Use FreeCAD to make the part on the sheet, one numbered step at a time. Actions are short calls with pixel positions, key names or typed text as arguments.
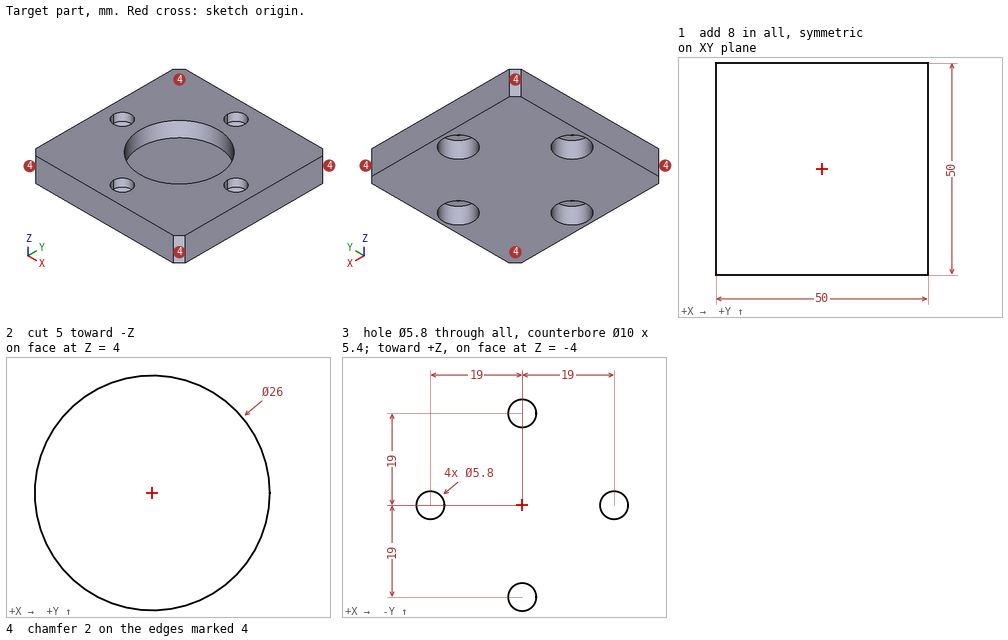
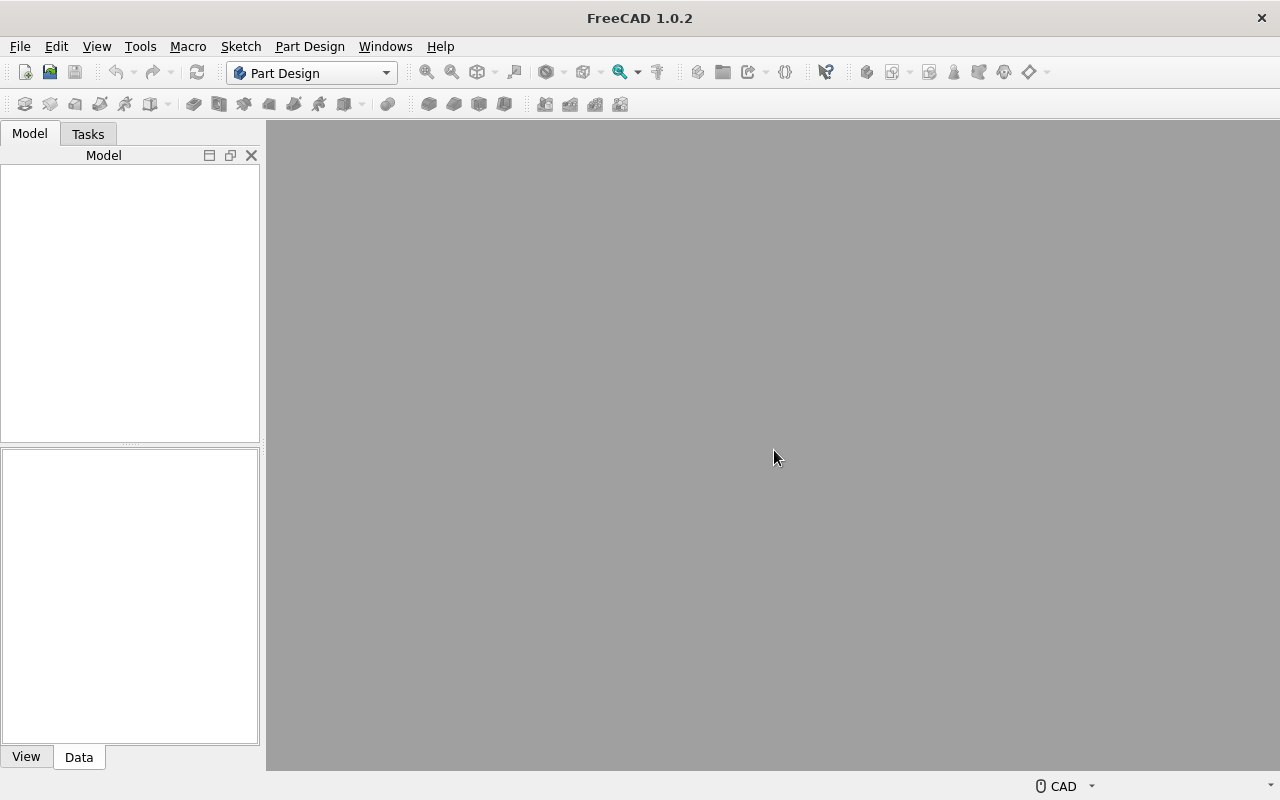
click(25, 72)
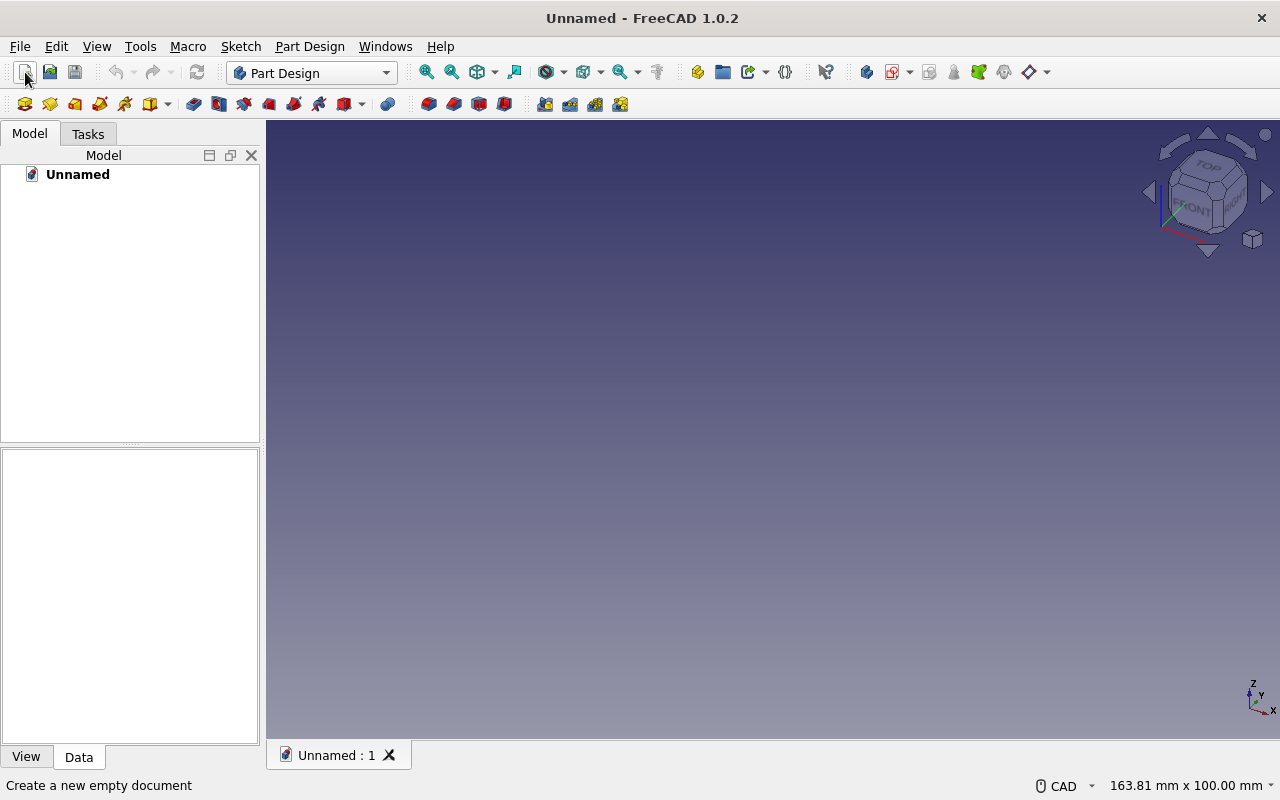
click(892, 72)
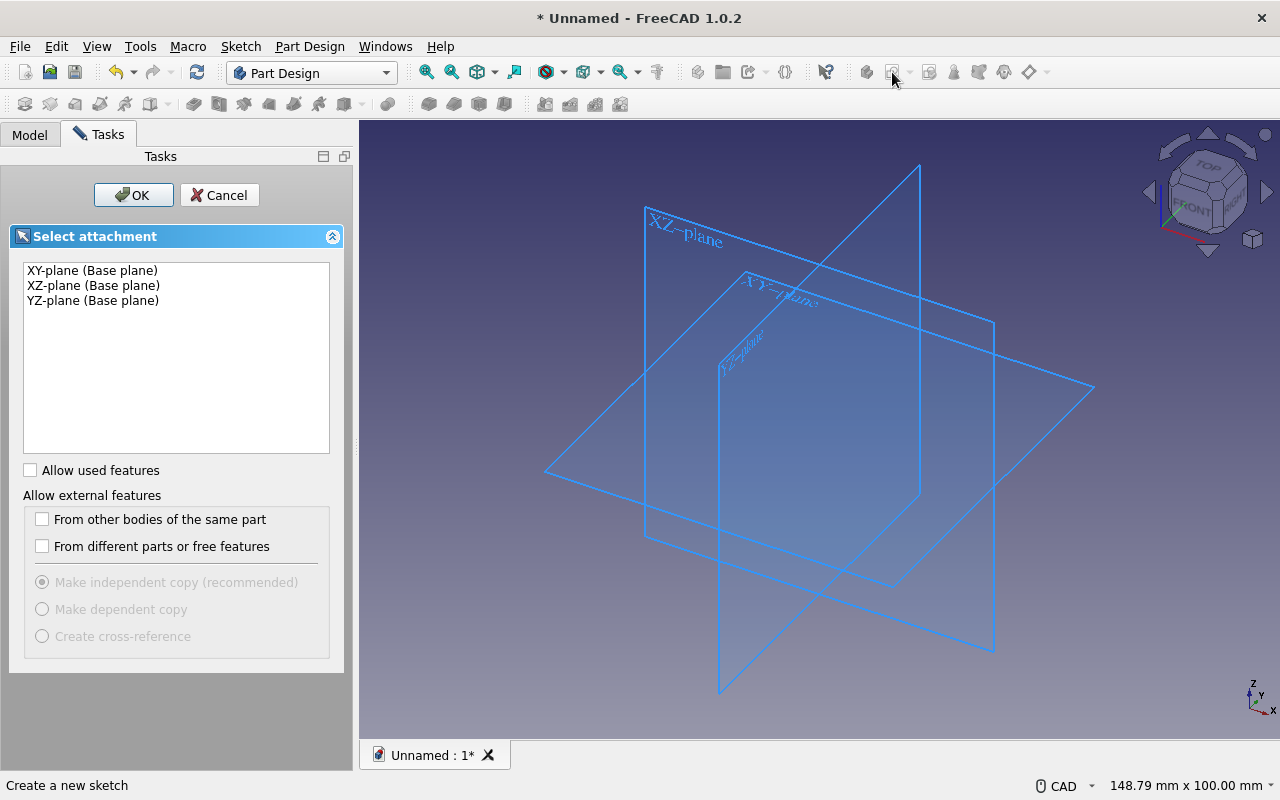
click(84, 270)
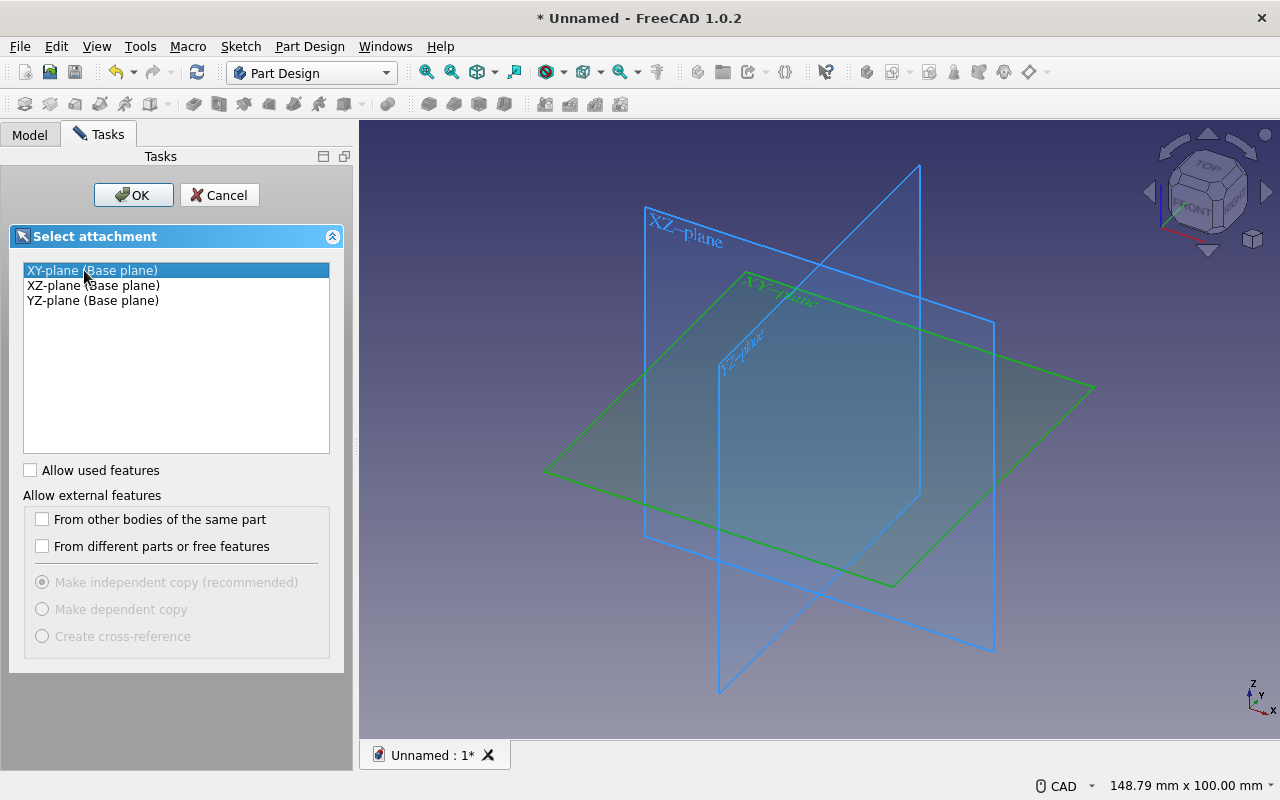
click(134, 195)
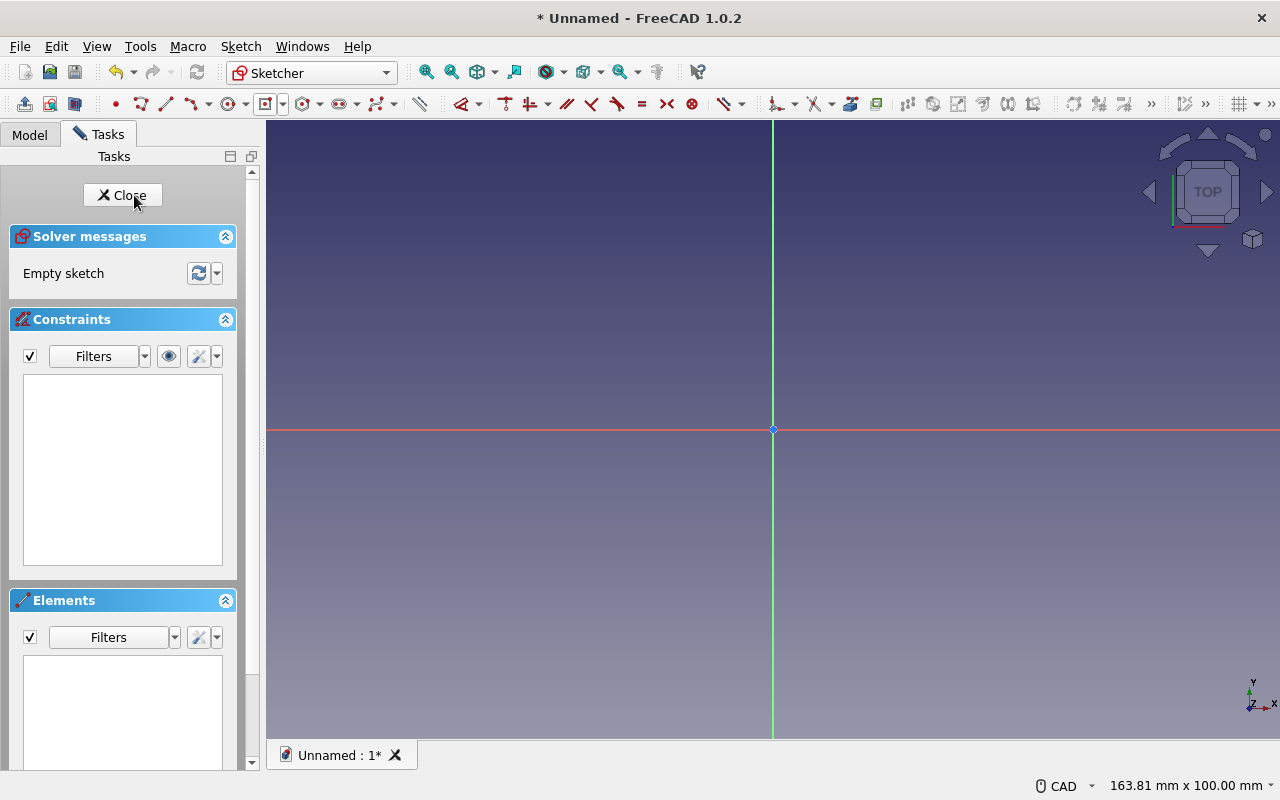
click(264, 104)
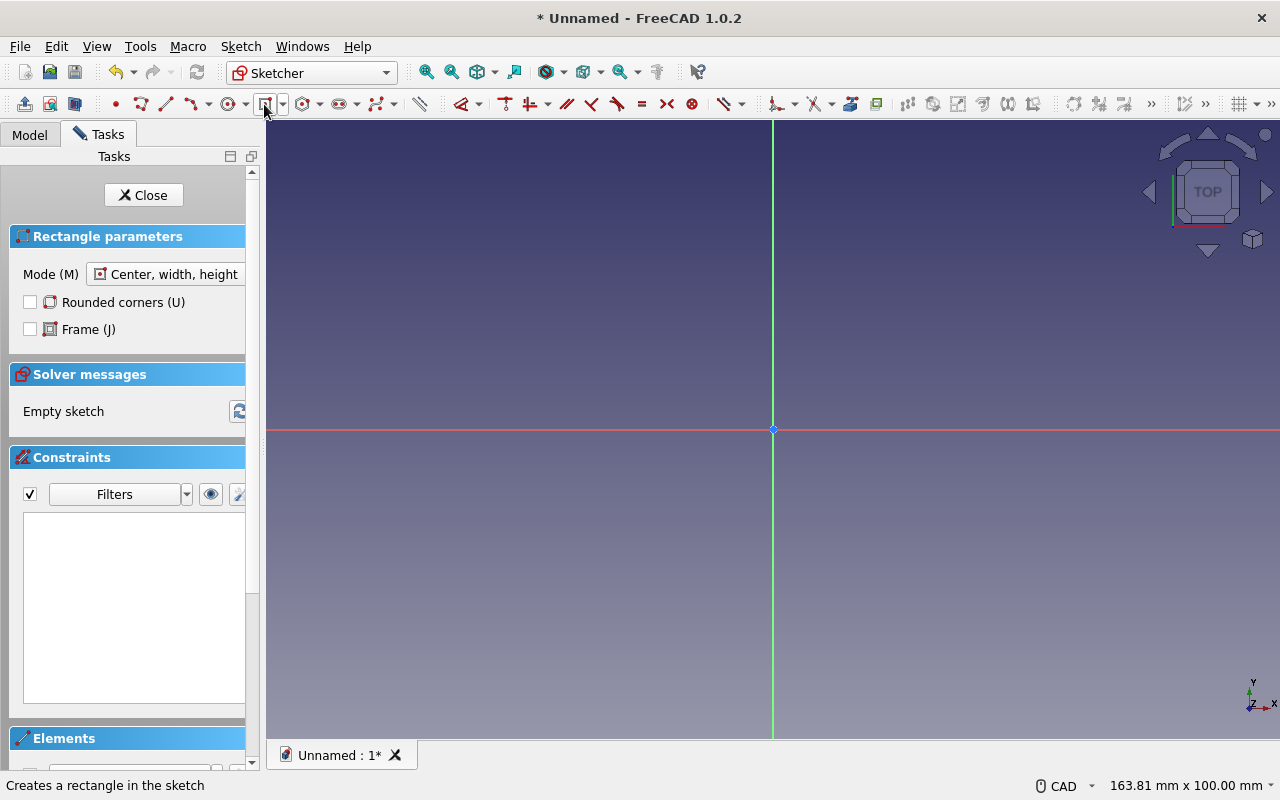
click(773, 430)
move(928, 275)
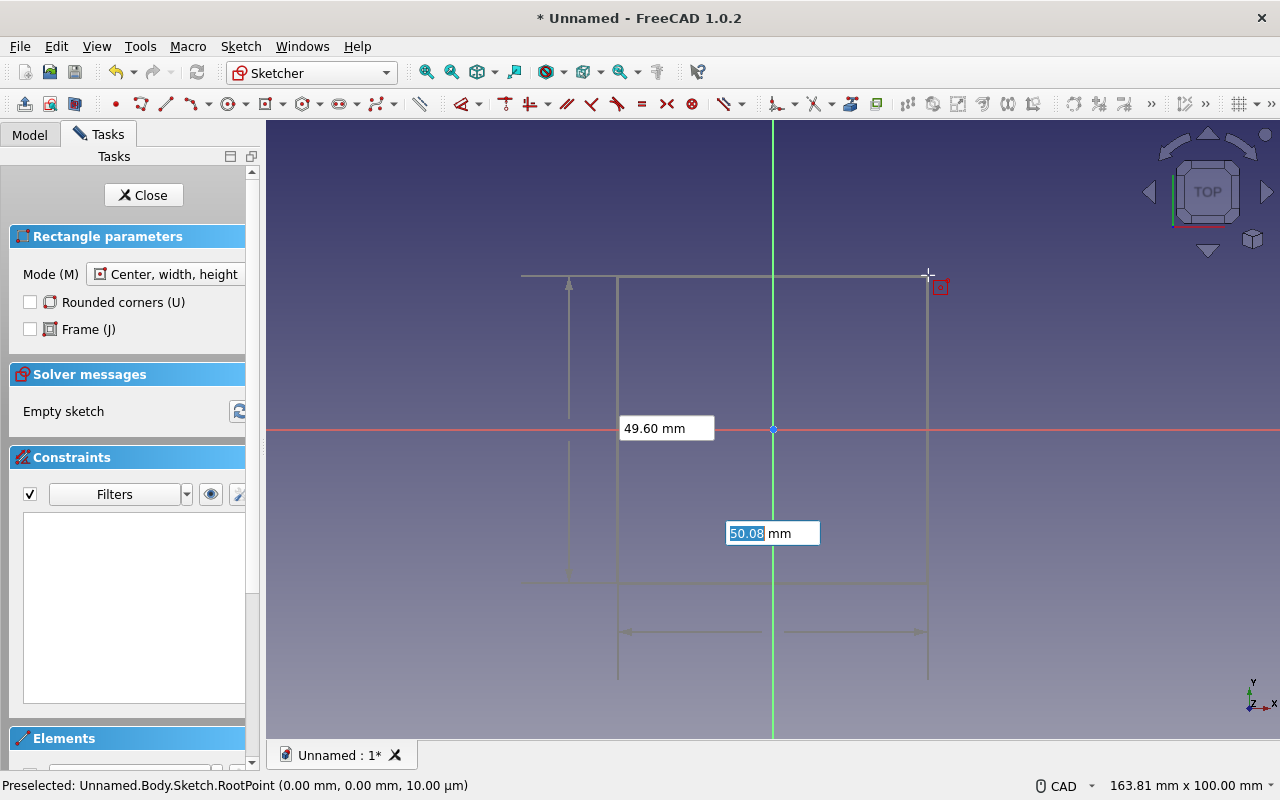
text(50)
key(Tab)
text(50)
key(Return)
key(Escape)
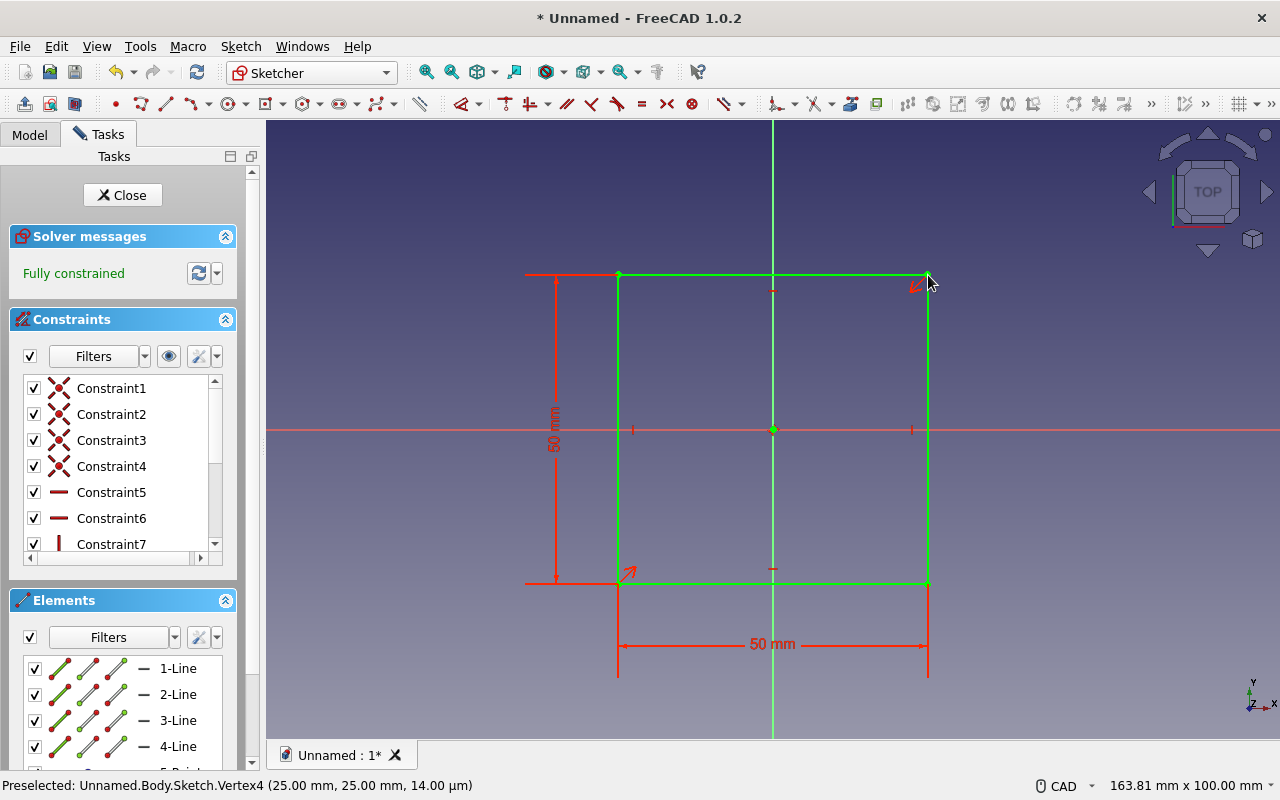
click(123, 195)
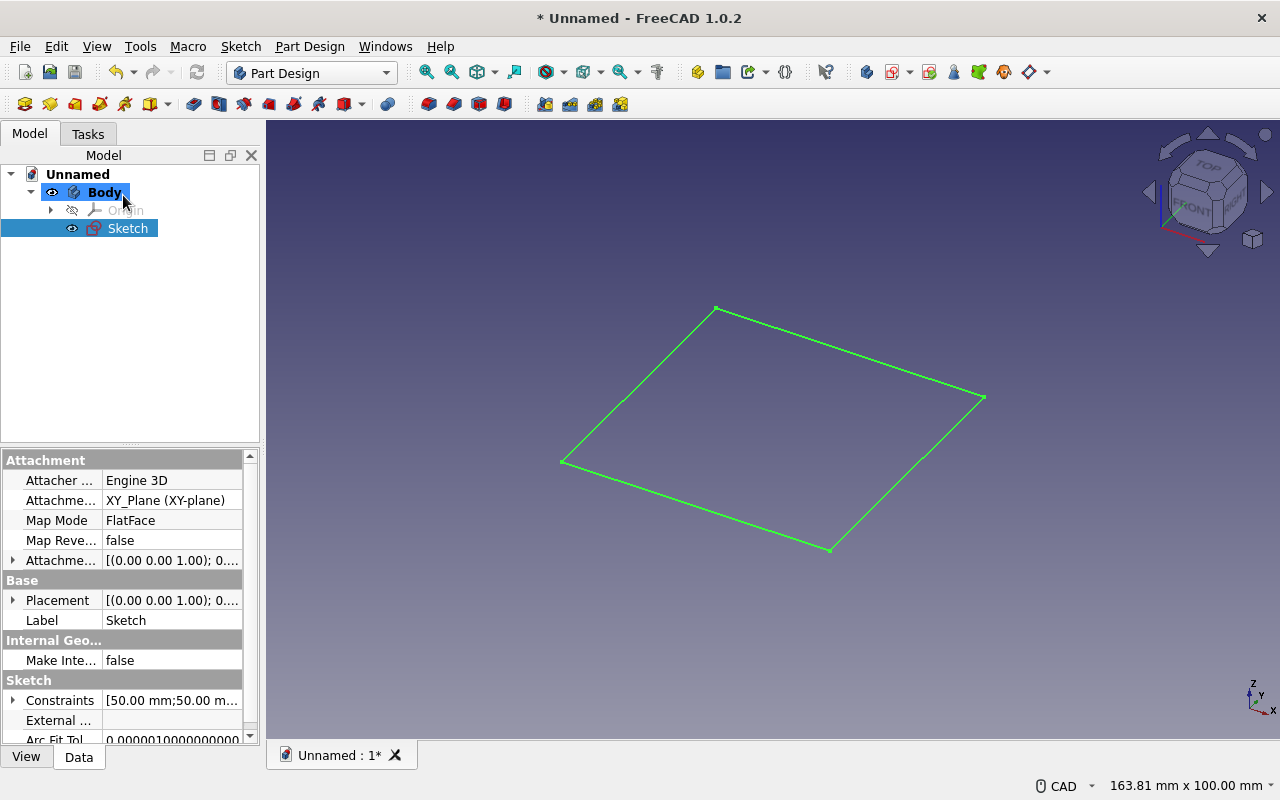
click(25, 104)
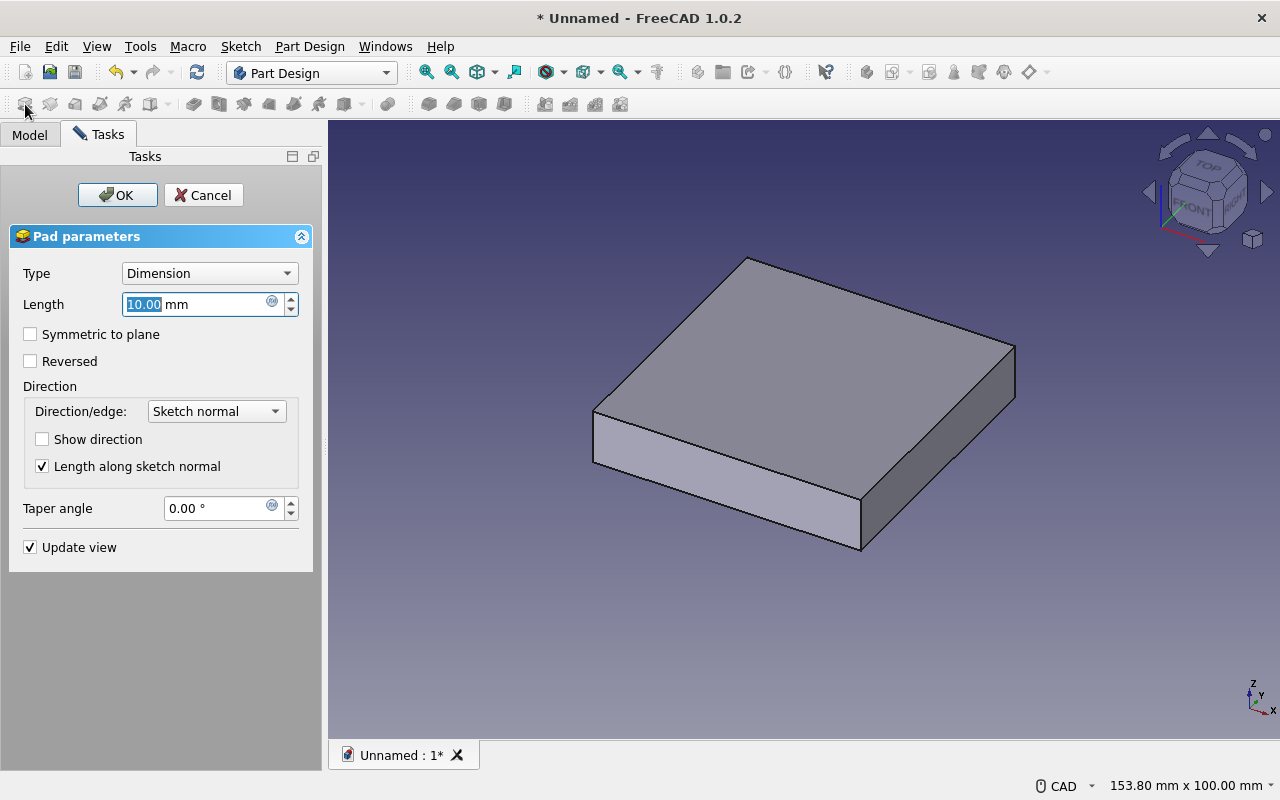
text(8)
key(Tab)